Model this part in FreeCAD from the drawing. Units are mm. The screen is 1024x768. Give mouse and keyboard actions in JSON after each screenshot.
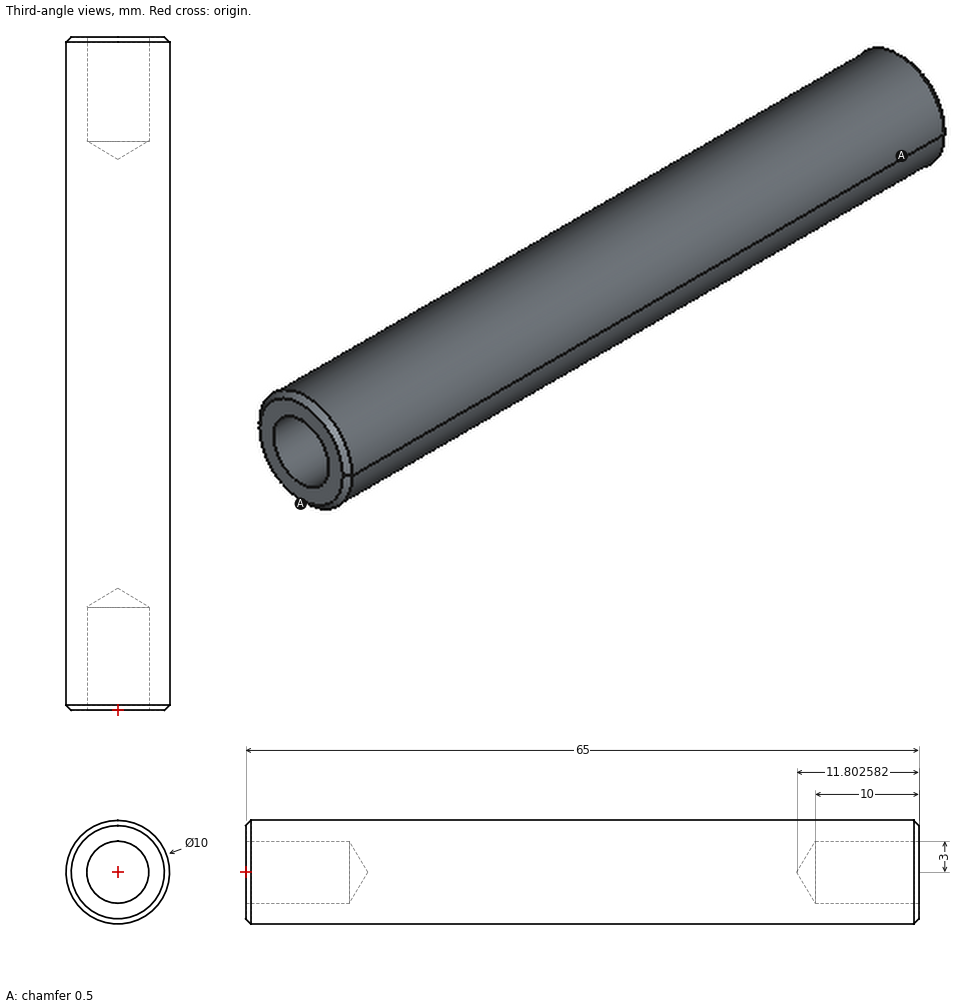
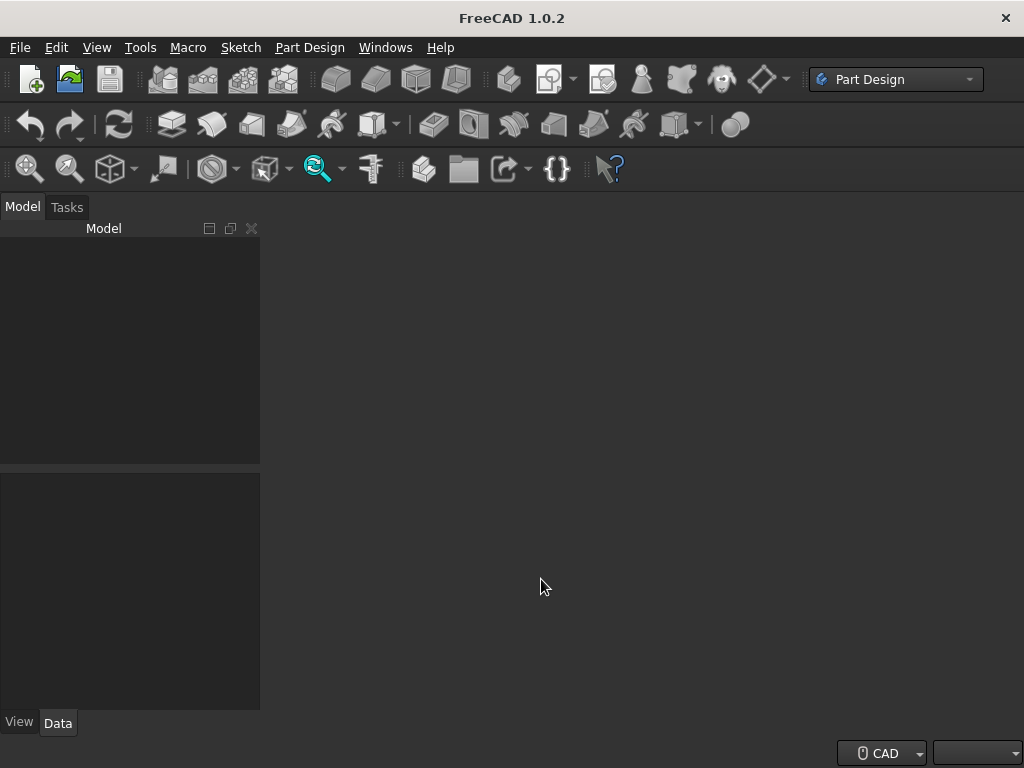
{"action": "left_click", "coordinate": [30, 80]}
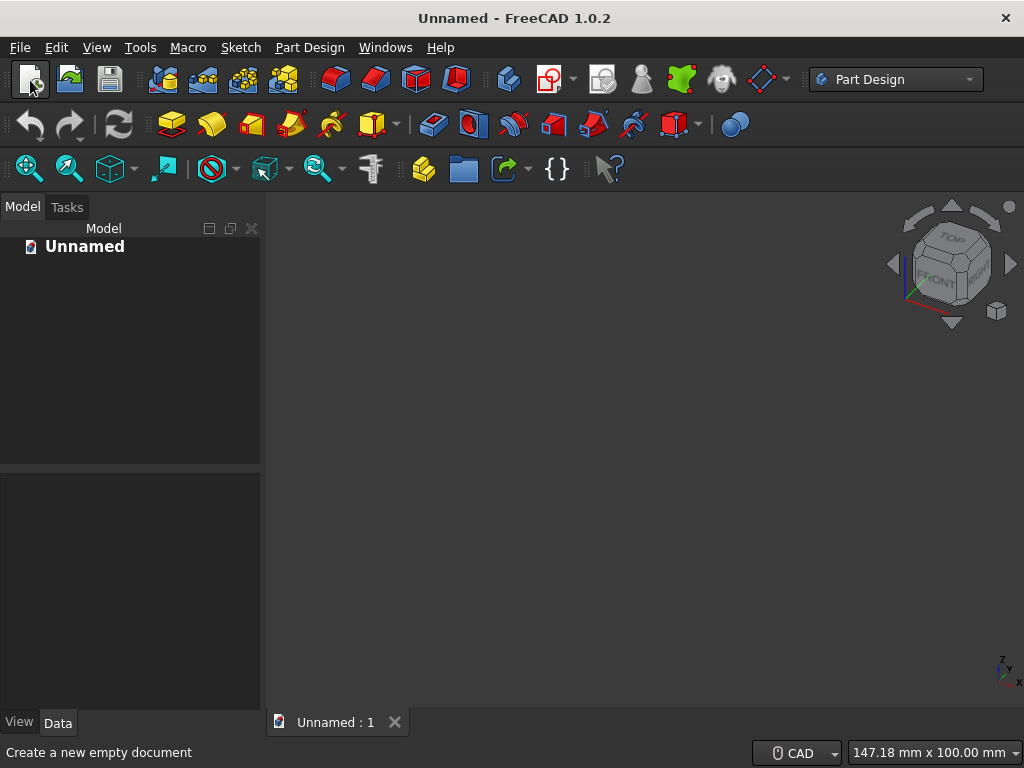
{"action": "left_click", "coordinate": [550, 80]}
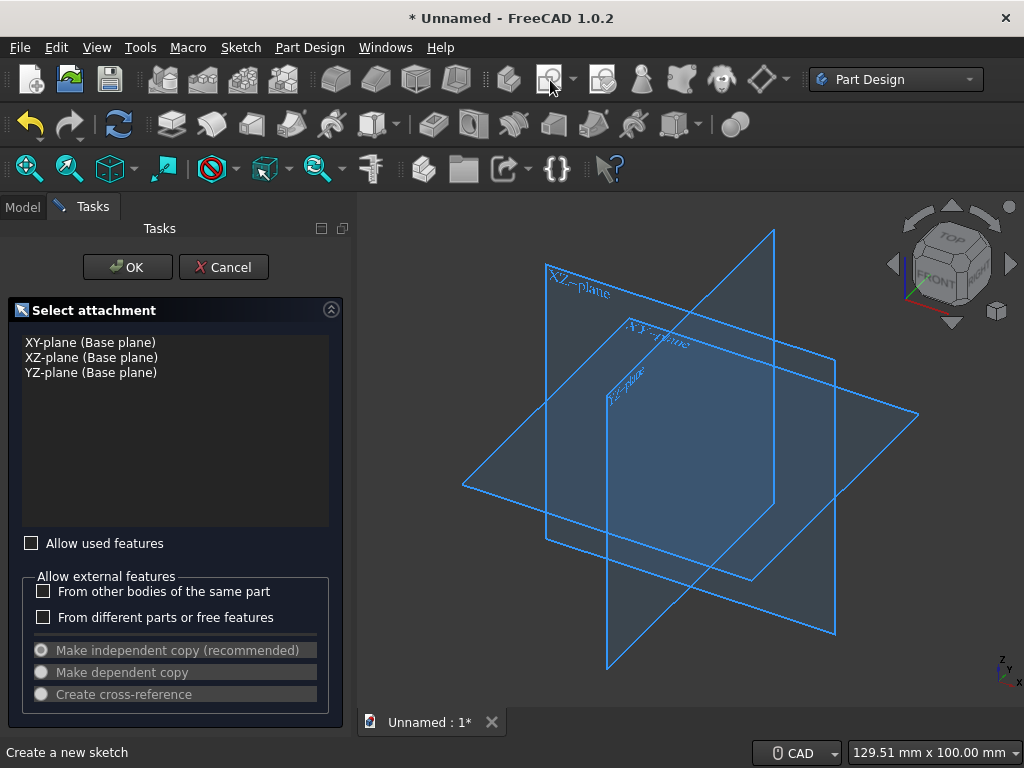
{"action": "left_click", "coordinate": [82, 358]}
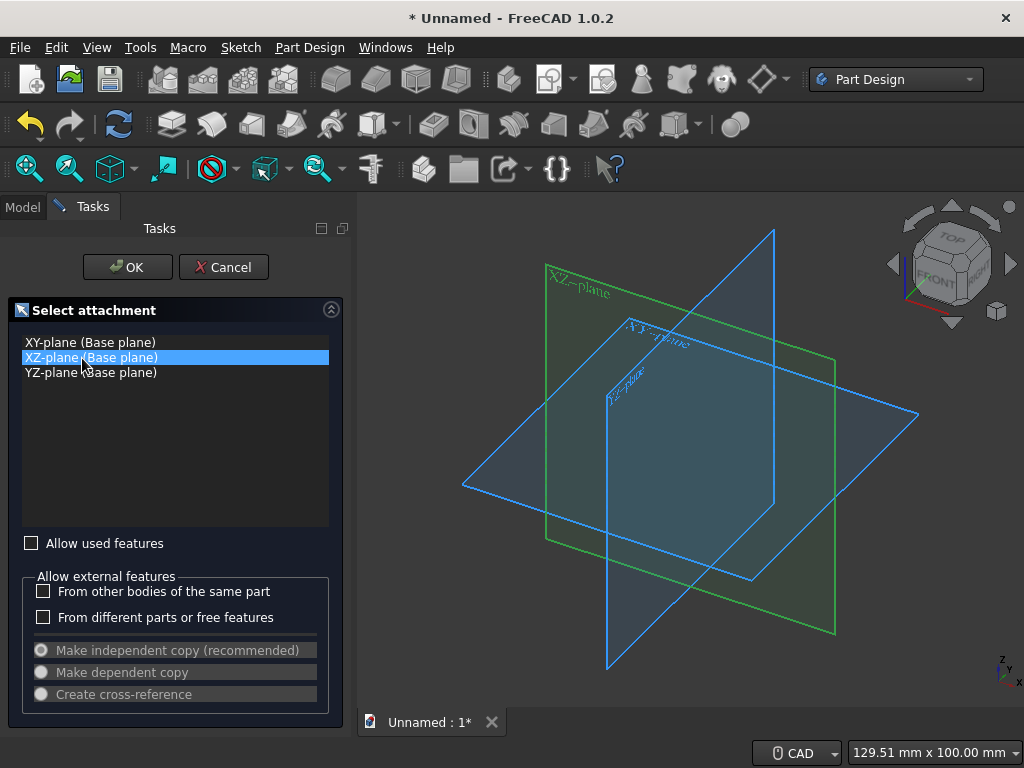
{"action": "left_click", "coordinate": [128, 267]}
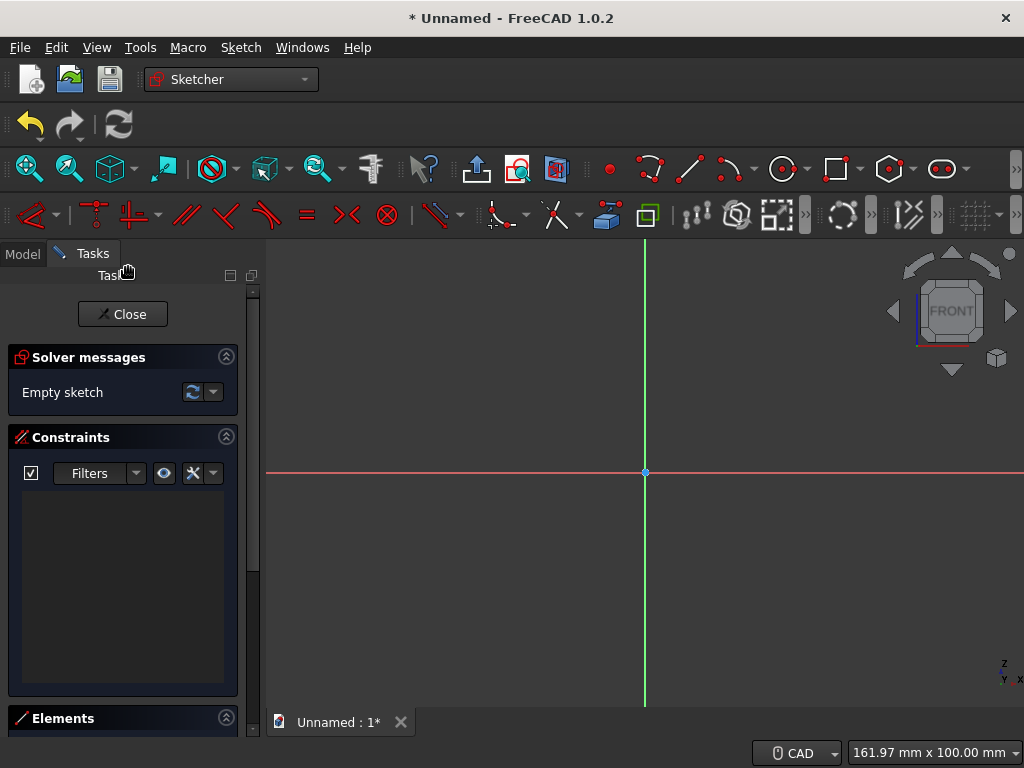
{"action": "scroll", "coordinate": [659, 473], "scroll_direction": "up", "scroll_amount": 9}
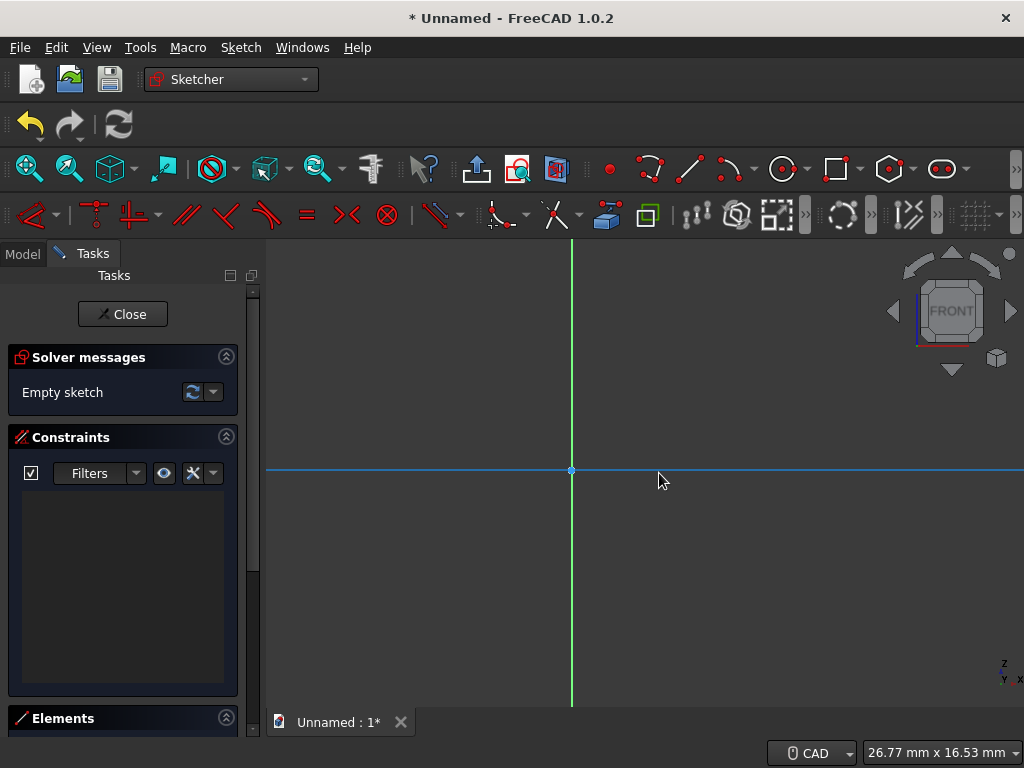
{"action": "left_click", "coordinate": [784, 170]}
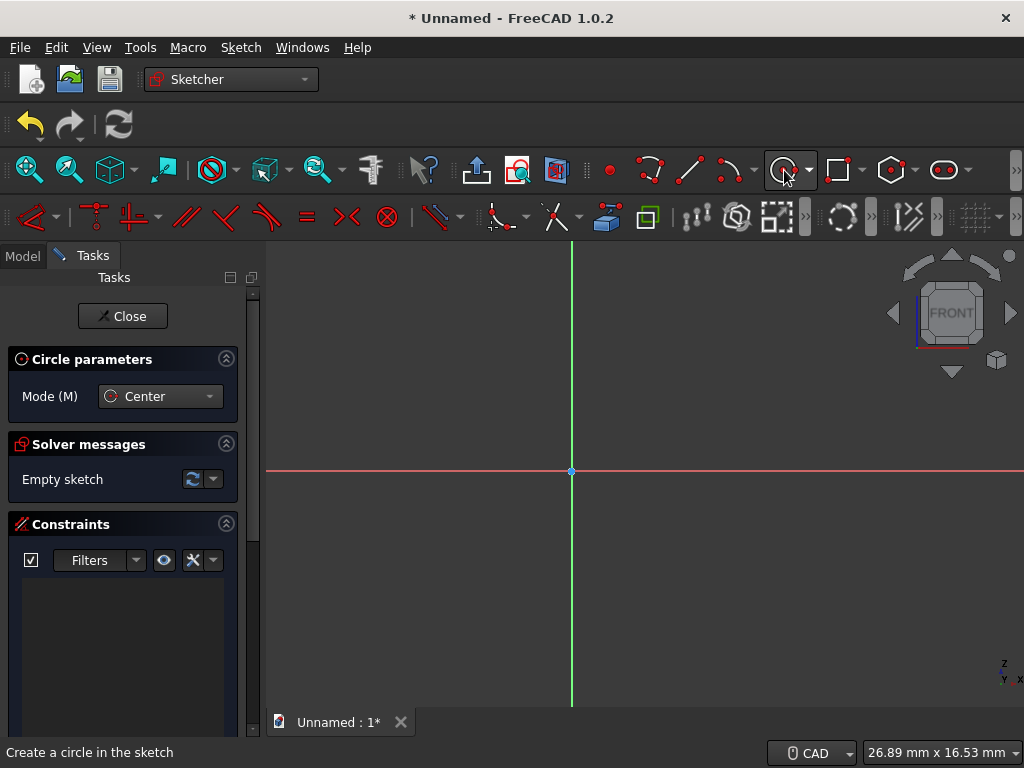
{"action": "left_click", "coordinate": [572, 471]}
{"action": "mouse_move", "coordinate": [672, 372]}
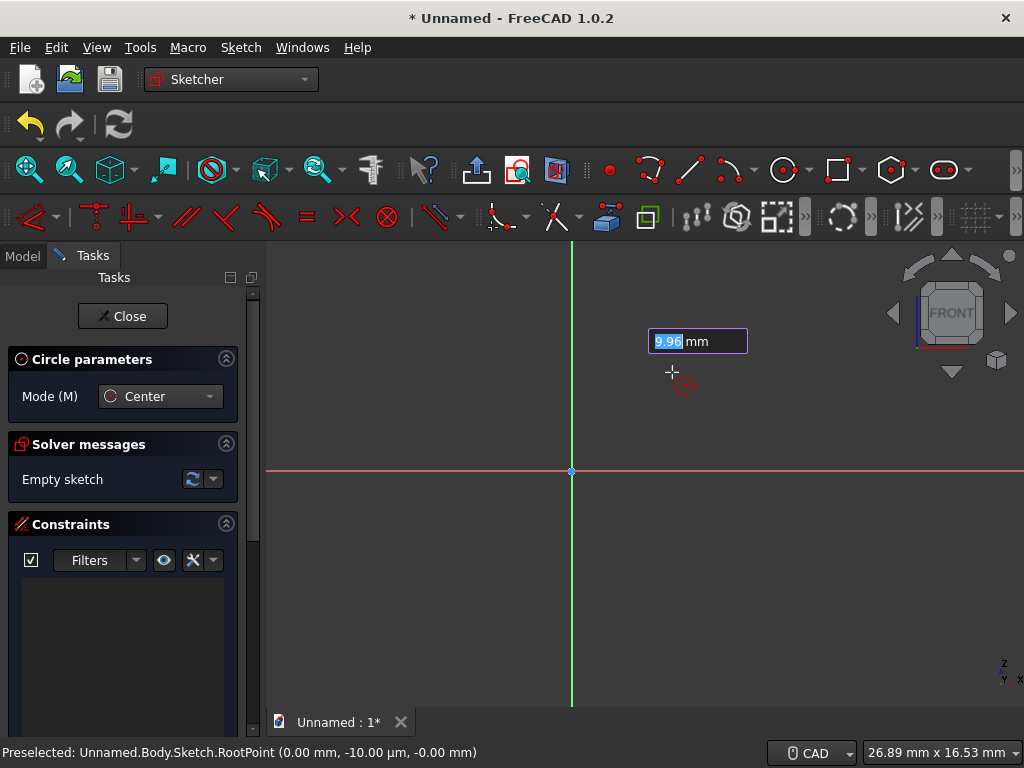
{"action": "type", "text": "10"}
{"action": "key", "text": "Return"}
{"action": "key", "text": "Escape"}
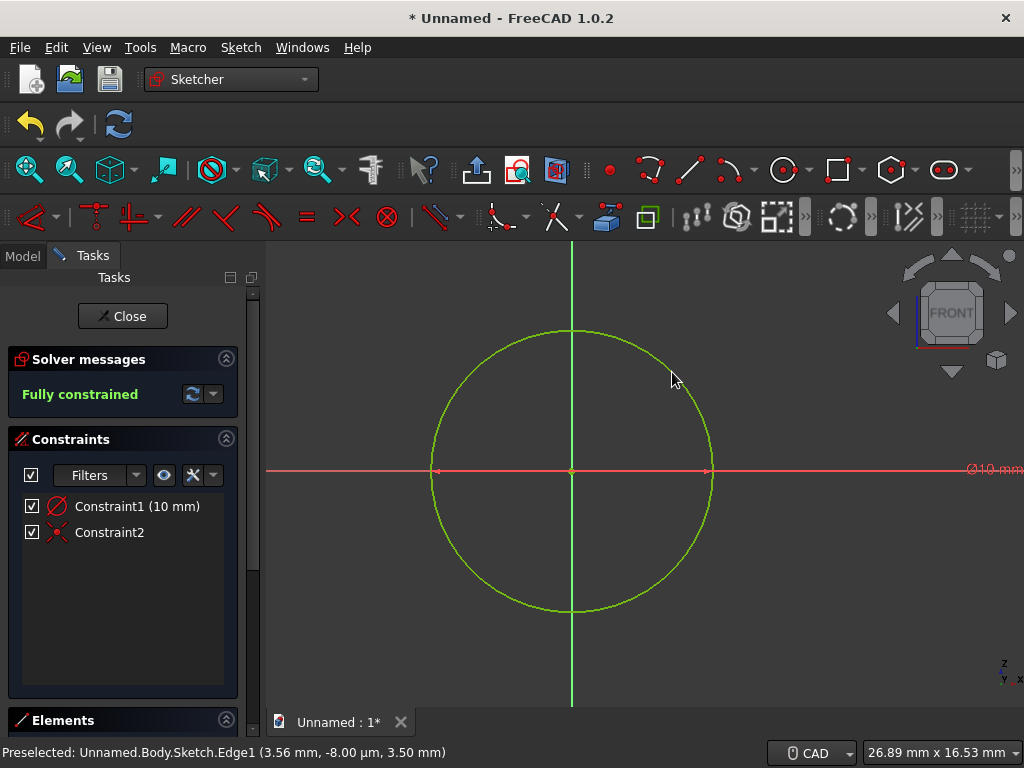
{"action": "left_click", "coordinate": [123, 316]}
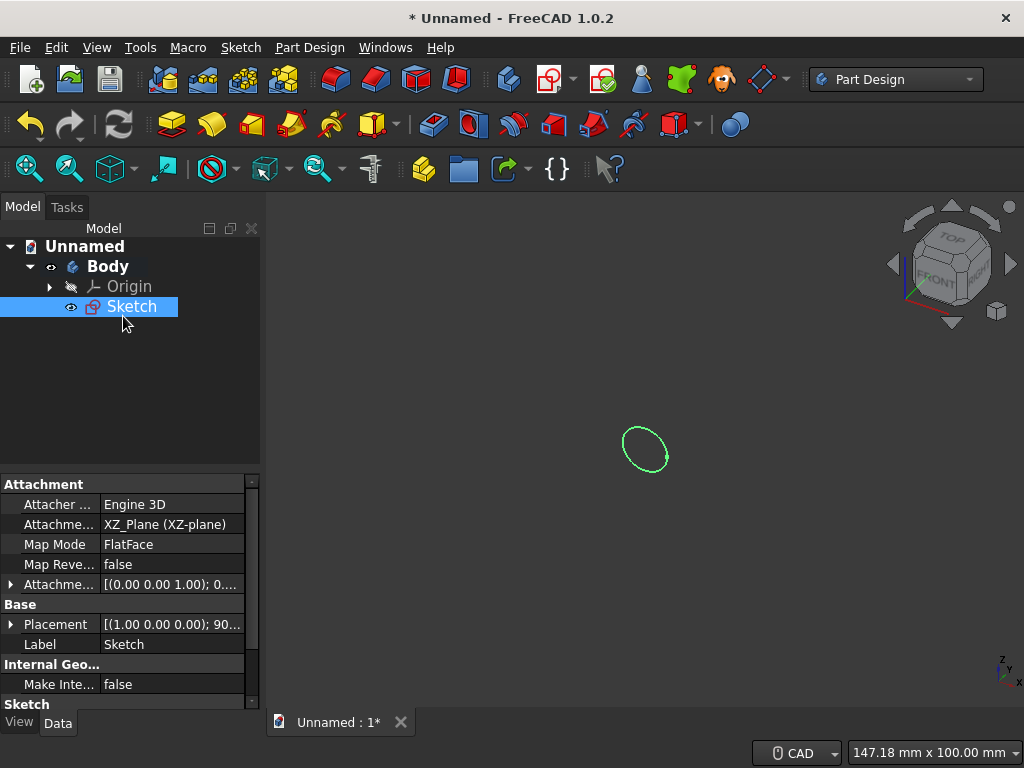
{"action": "left_click", "coordinate": [172, 124]}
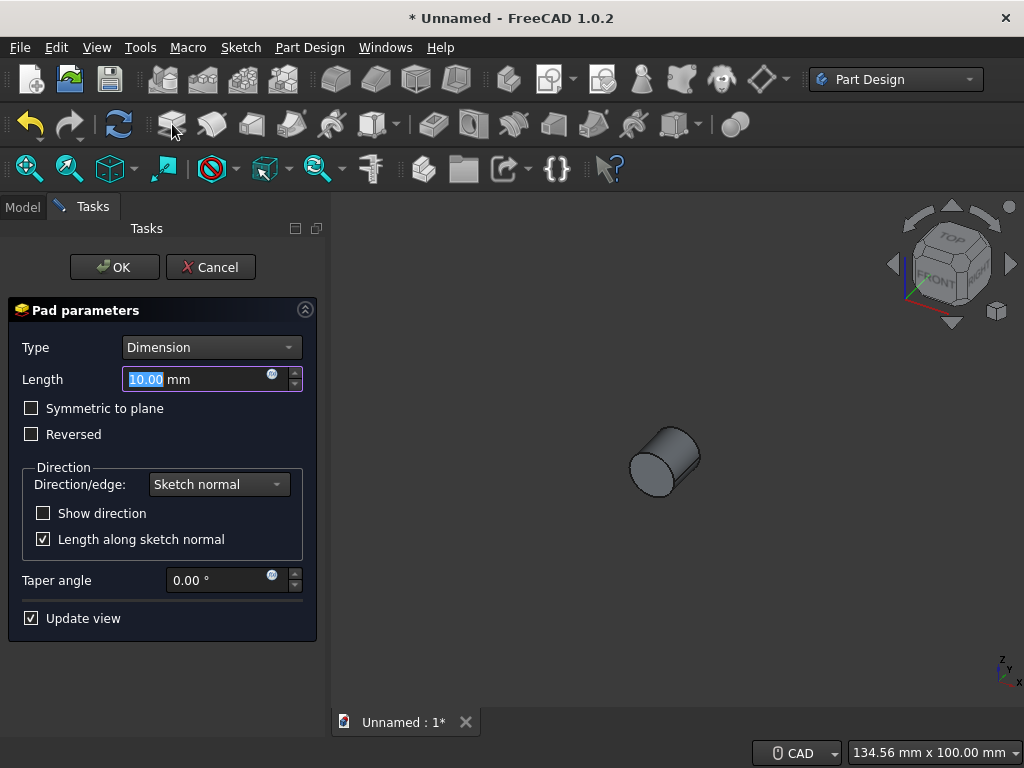
{"action": "type", "text": "65"}
{"action": "key", "text": "Tab"}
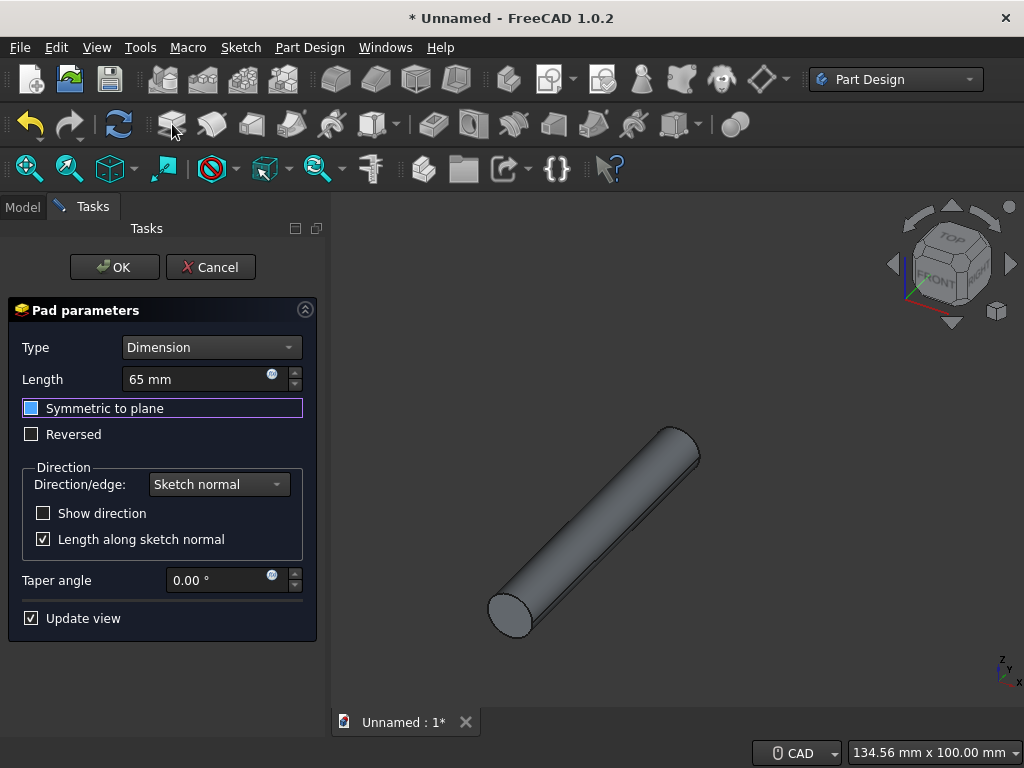
{"action": "left_click", "coordinate": [30, 434]}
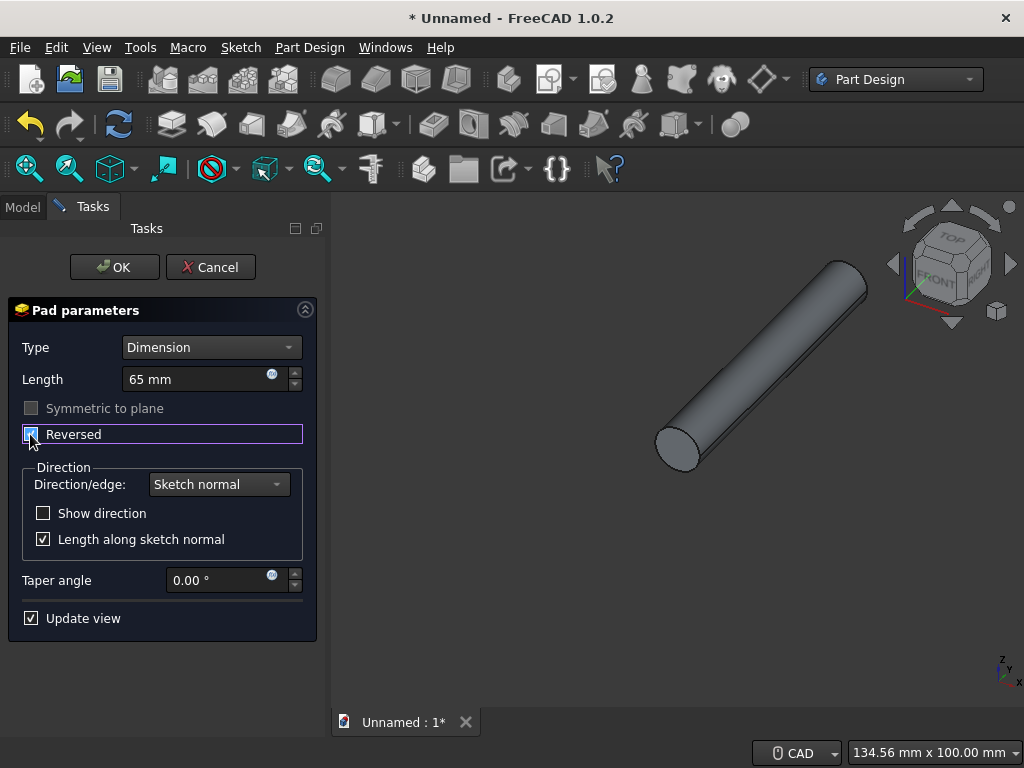
{"action": "left_click", "coordinate": [115, 267]}